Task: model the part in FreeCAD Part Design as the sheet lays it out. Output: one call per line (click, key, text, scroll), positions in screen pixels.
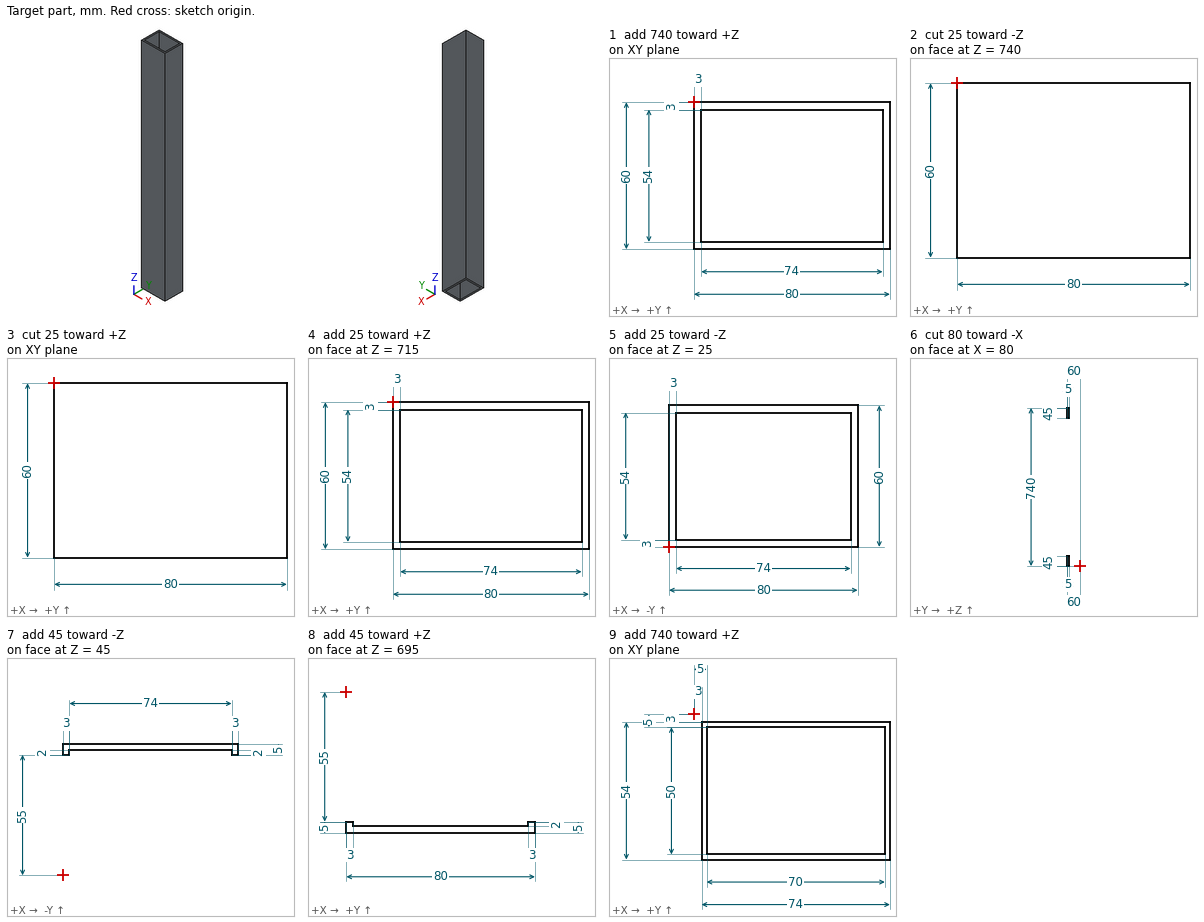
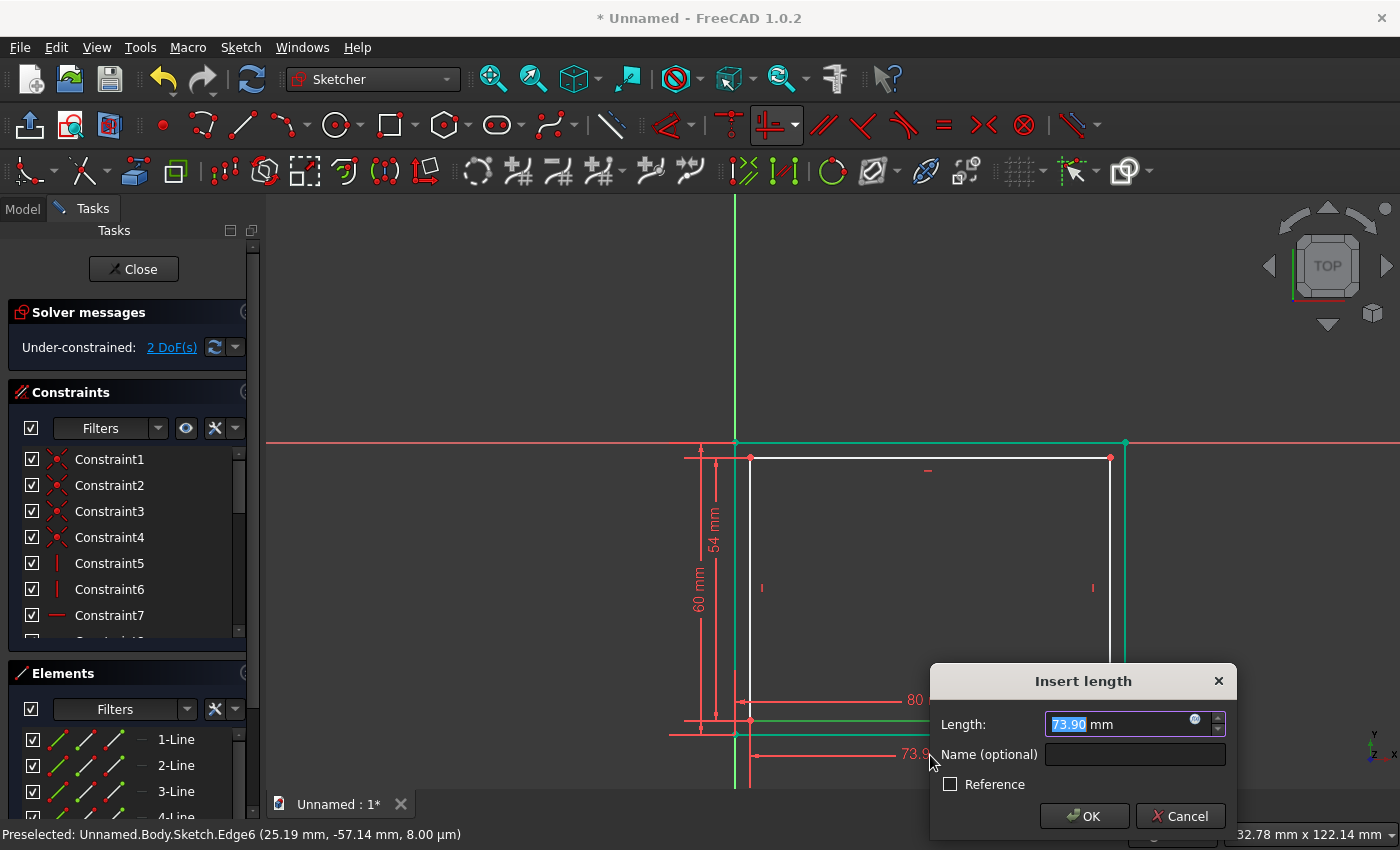
text(74)
key(Return)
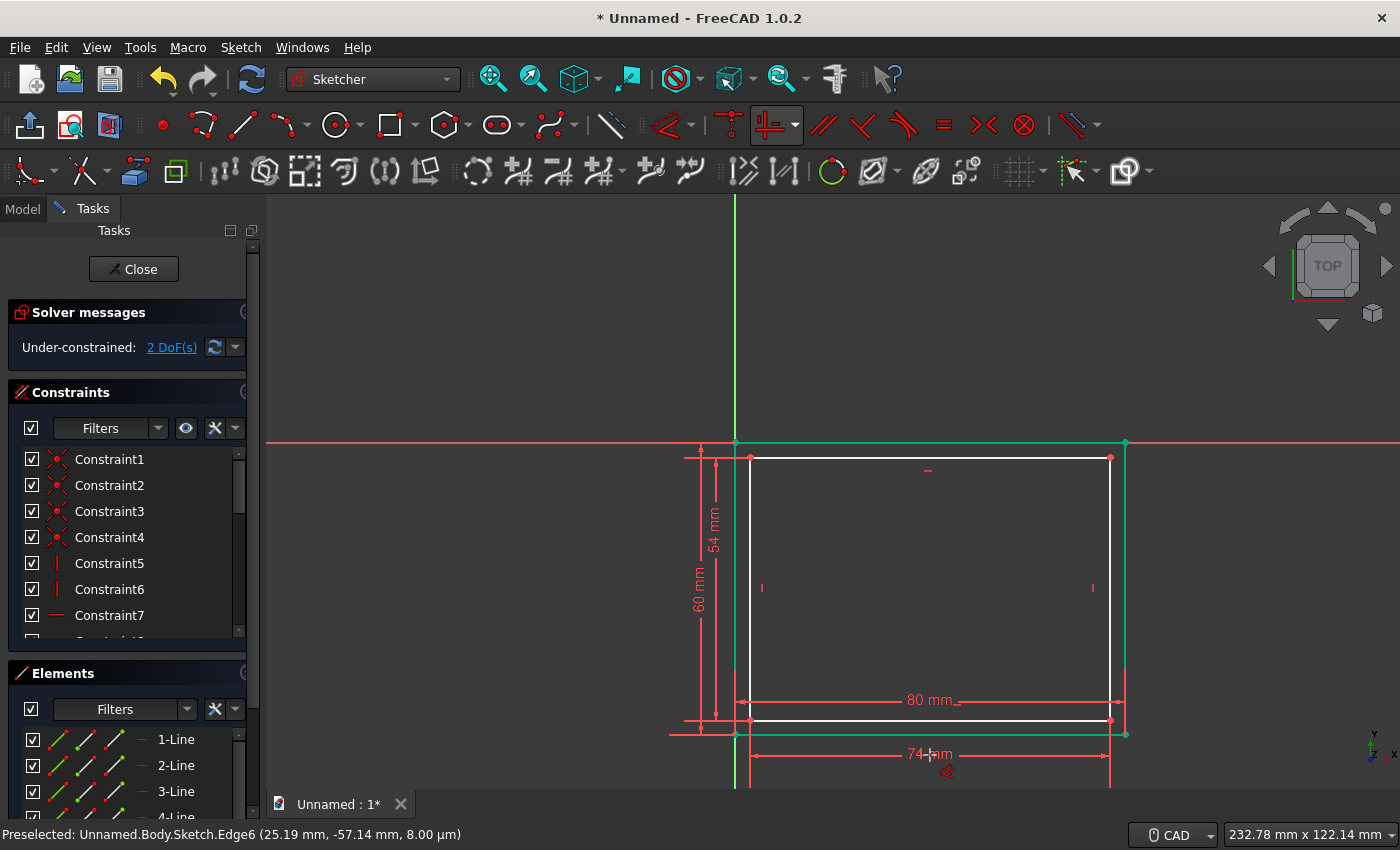
scroll(750, 458, up, 5)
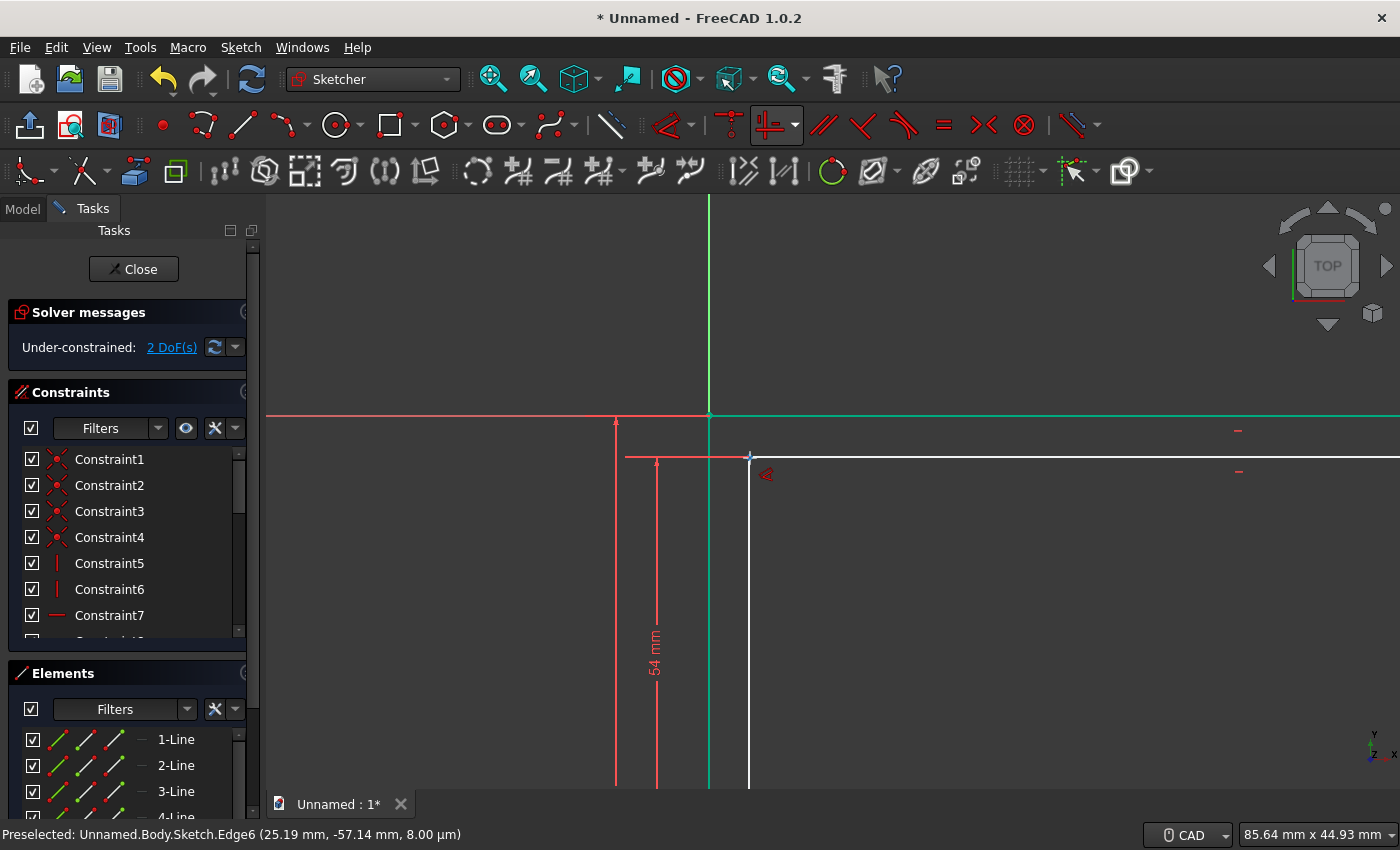
click(749, 457)
click(729, 382)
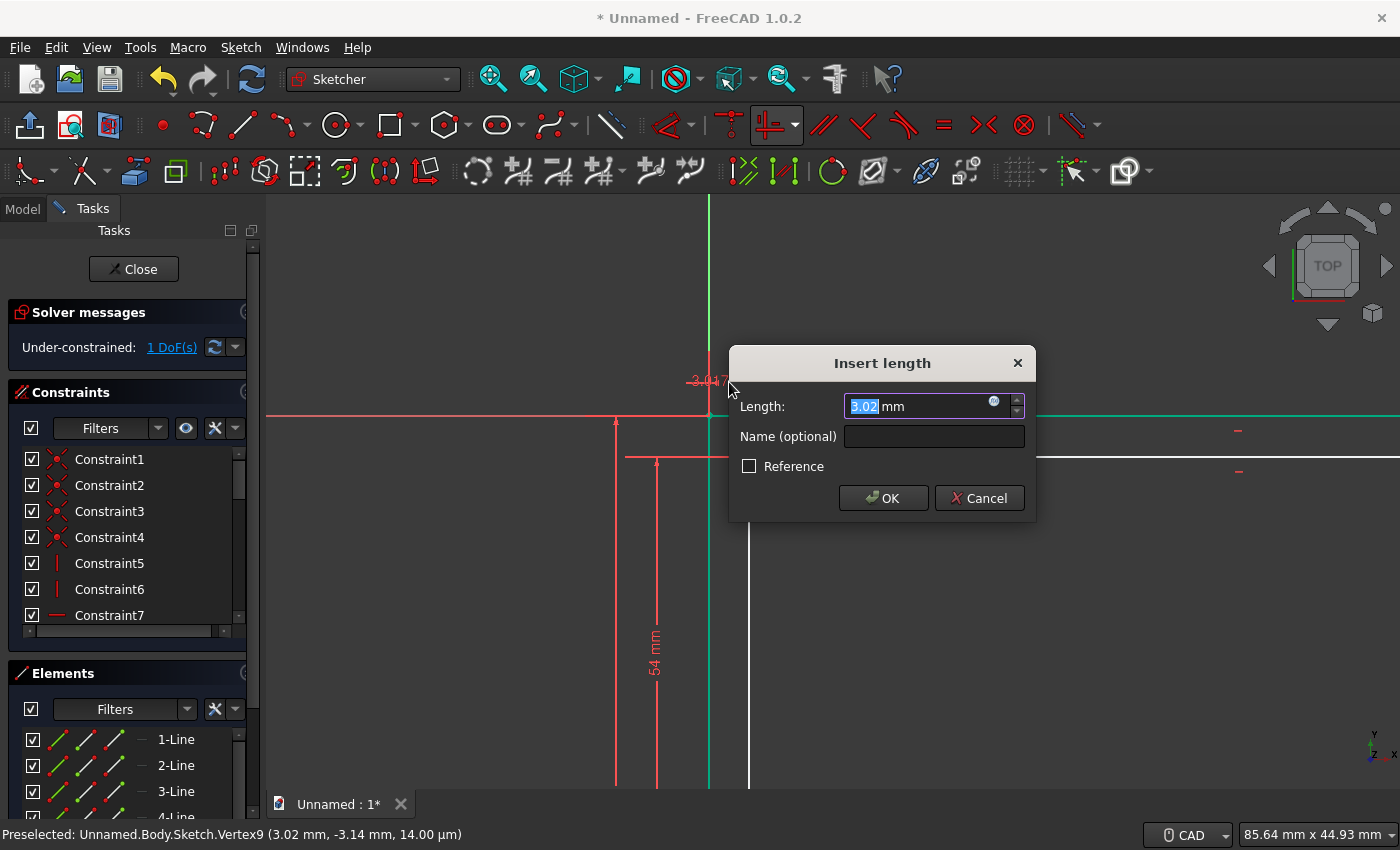
text(3)
key(Return)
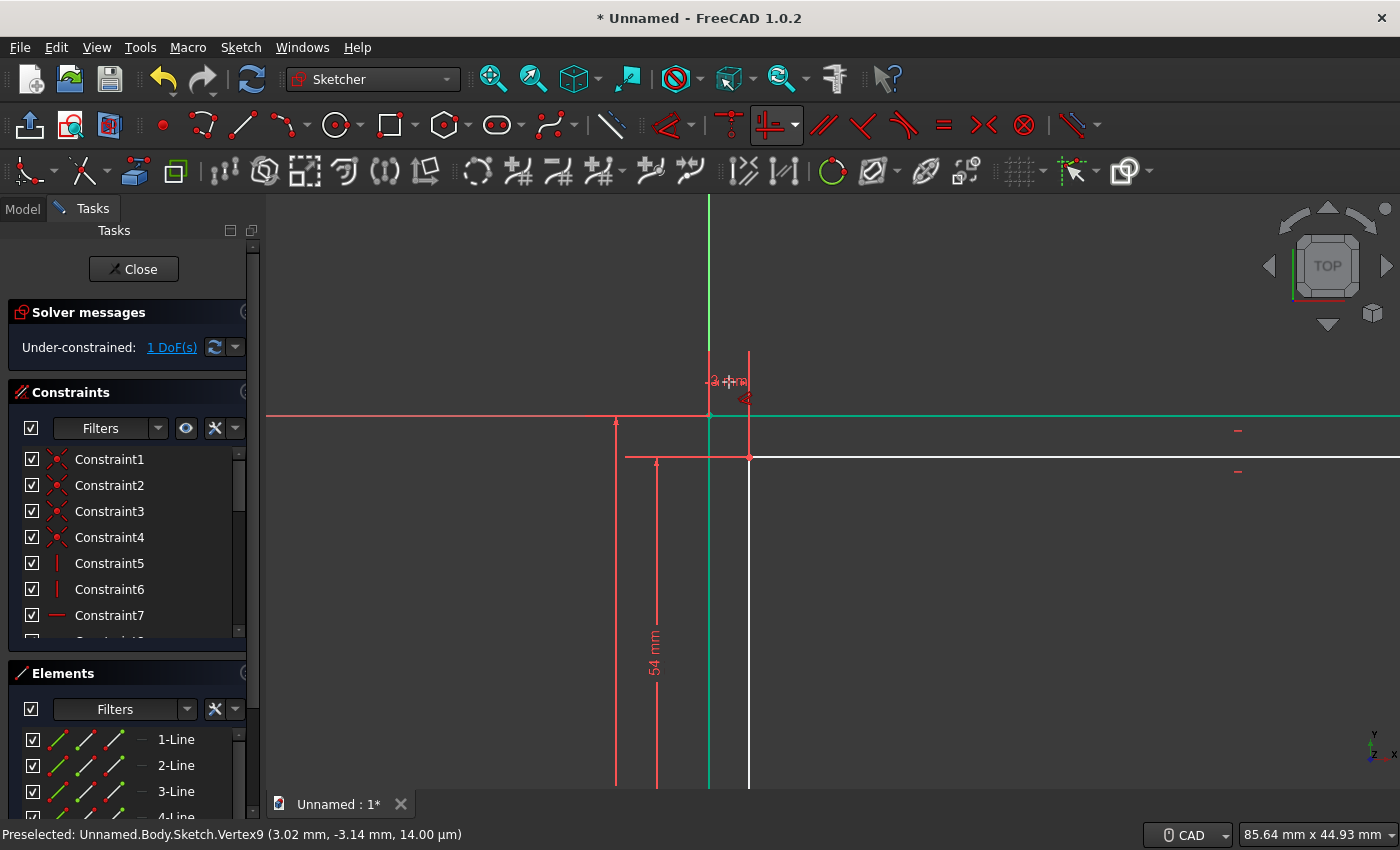
click(749, 457)
click(675, 436)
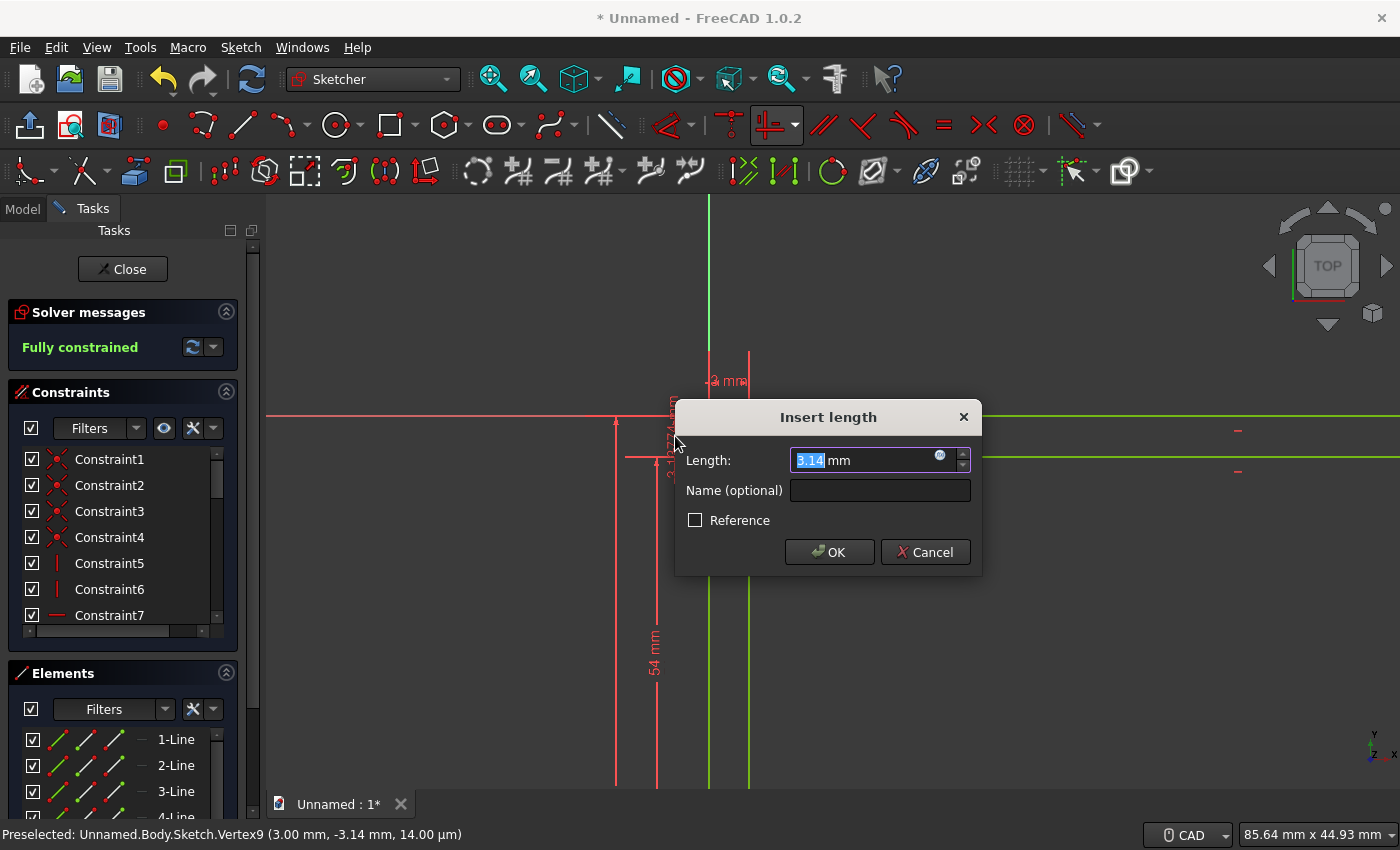
text(3)
key(Return)
key(Escape)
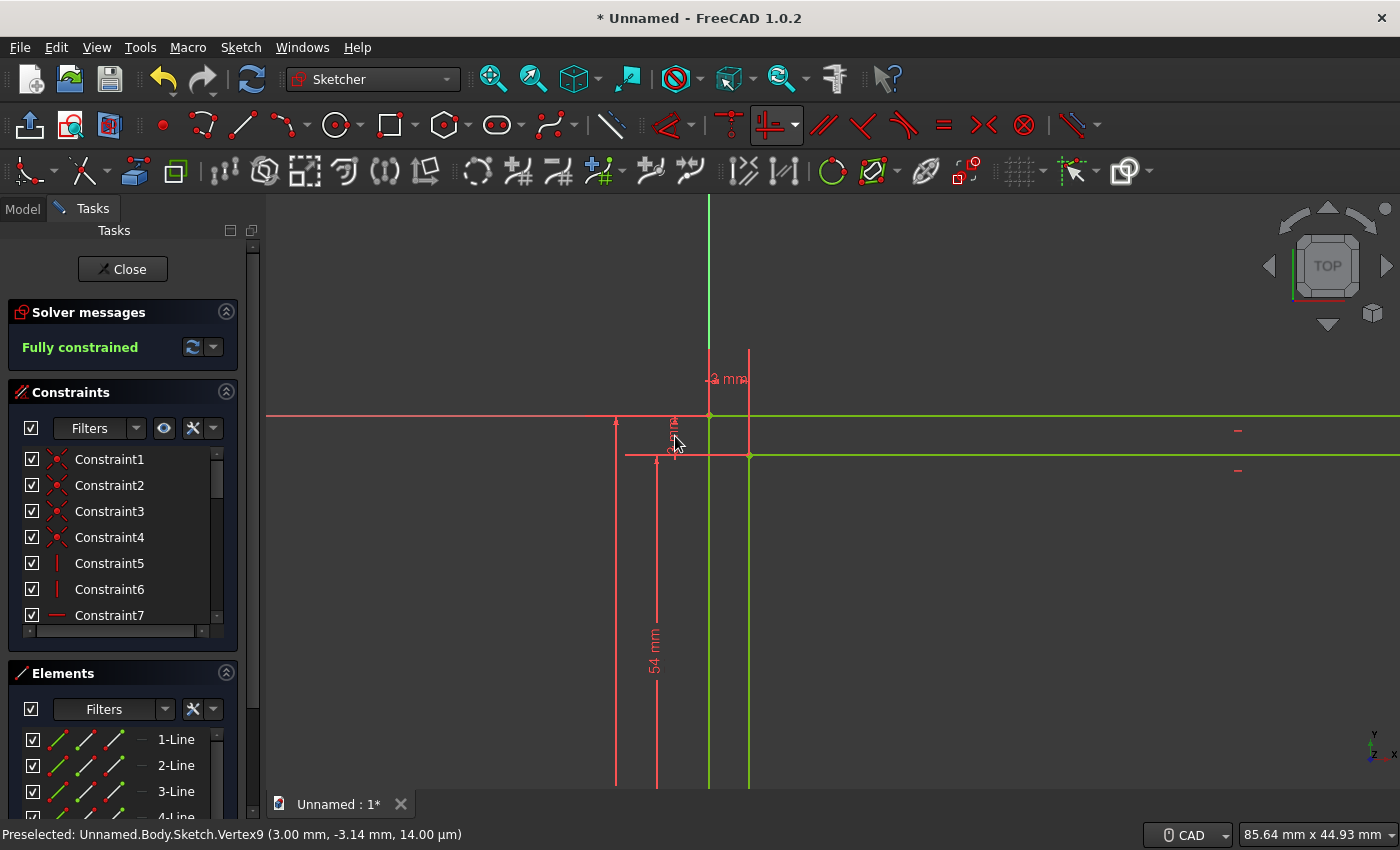
click(123, 269)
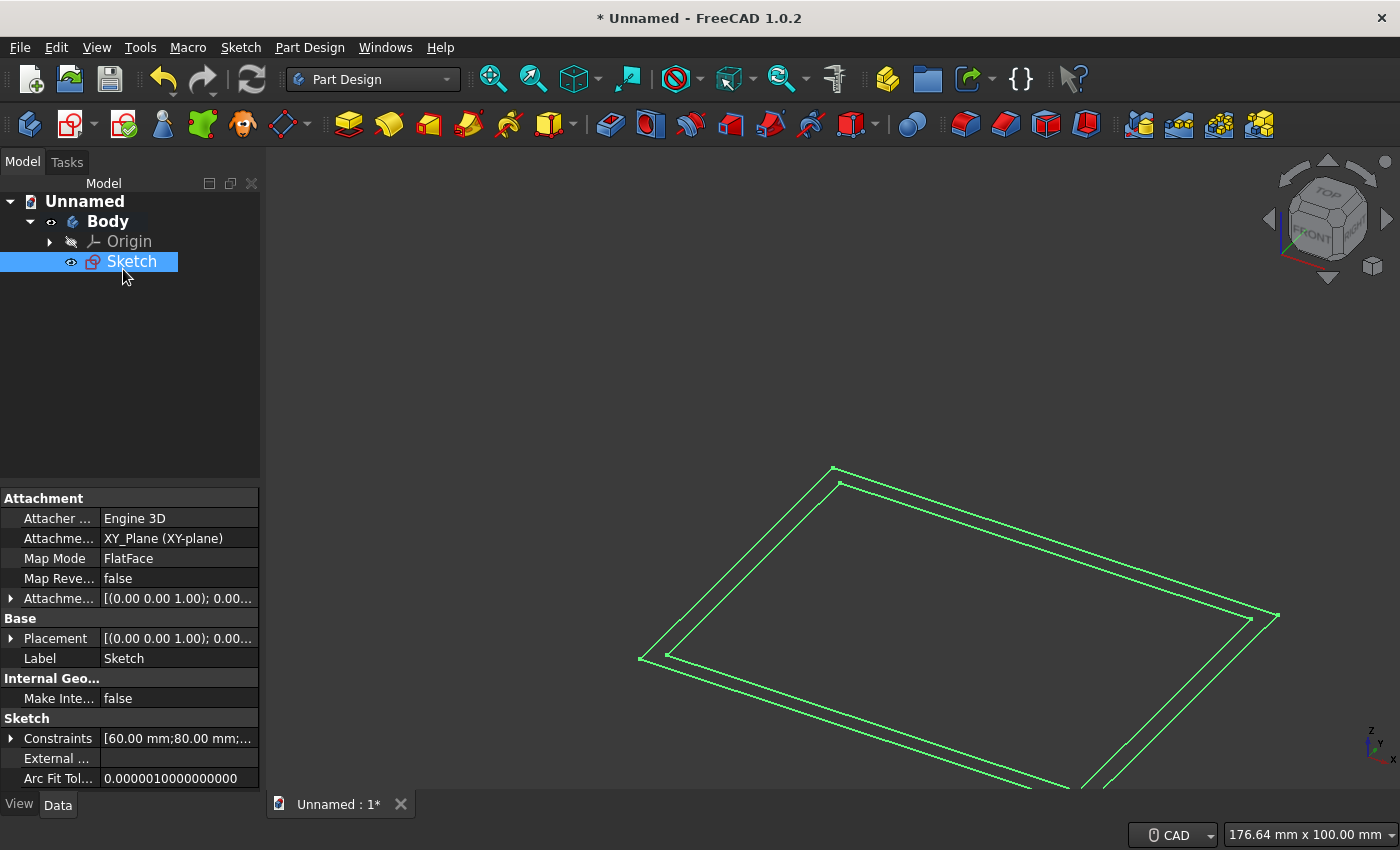
click(350, 124)